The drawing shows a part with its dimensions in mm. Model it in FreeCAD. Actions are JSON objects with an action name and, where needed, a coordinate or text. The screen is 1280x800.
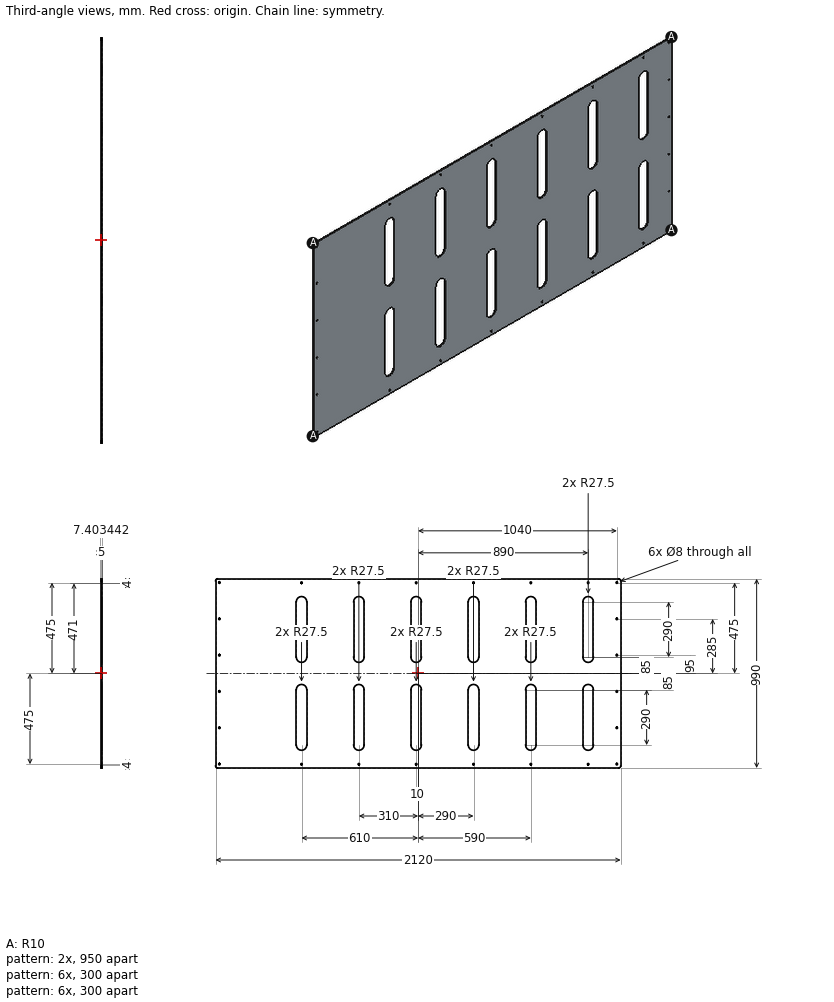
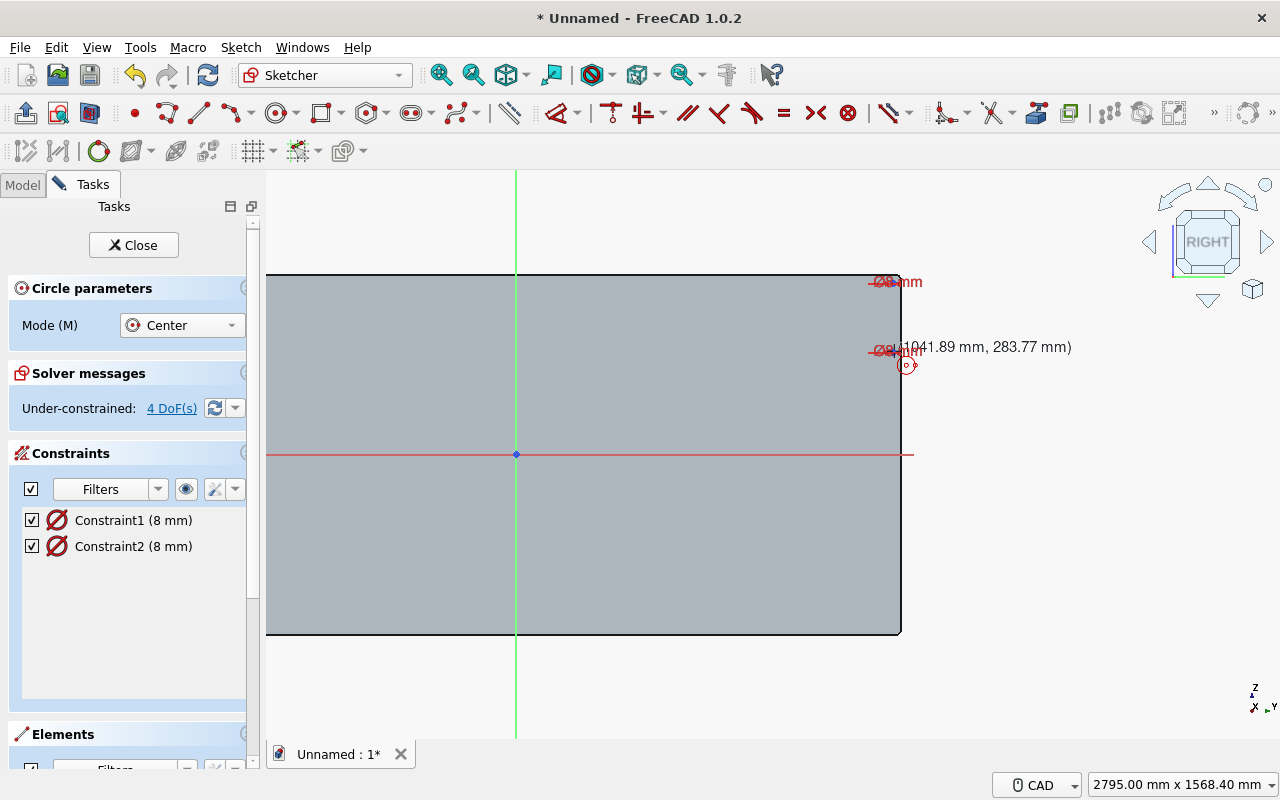
{"action": "scroll", "coordinate": [893, 420], "scroll_direction": "up", "scroll_amount": 14}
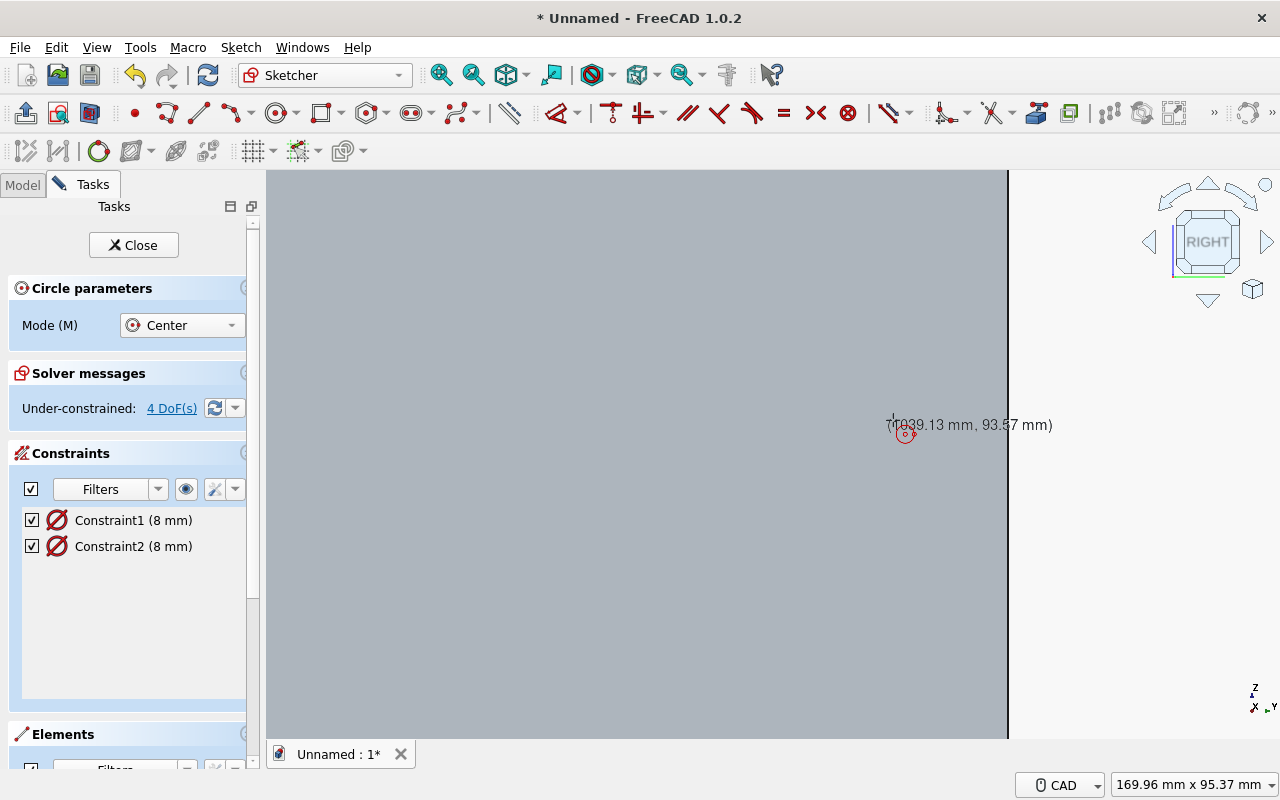
{"action": "scroll", "coordinate": [893, 420], "scroll_direction": "down", "scroll_amount": 14}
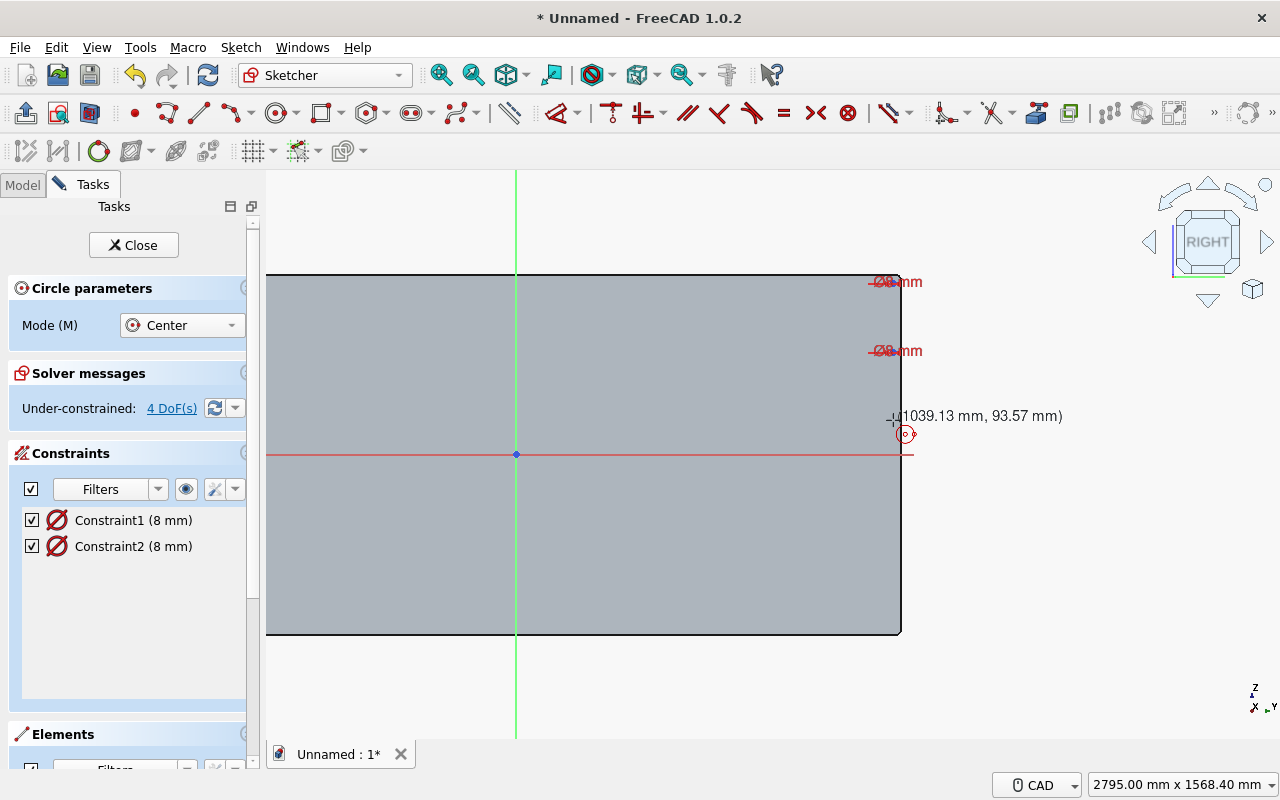
{"action": "left_click", "coordinate": [893, 420]}
{"action": "mouse_move", "coordinate": [894, 419]}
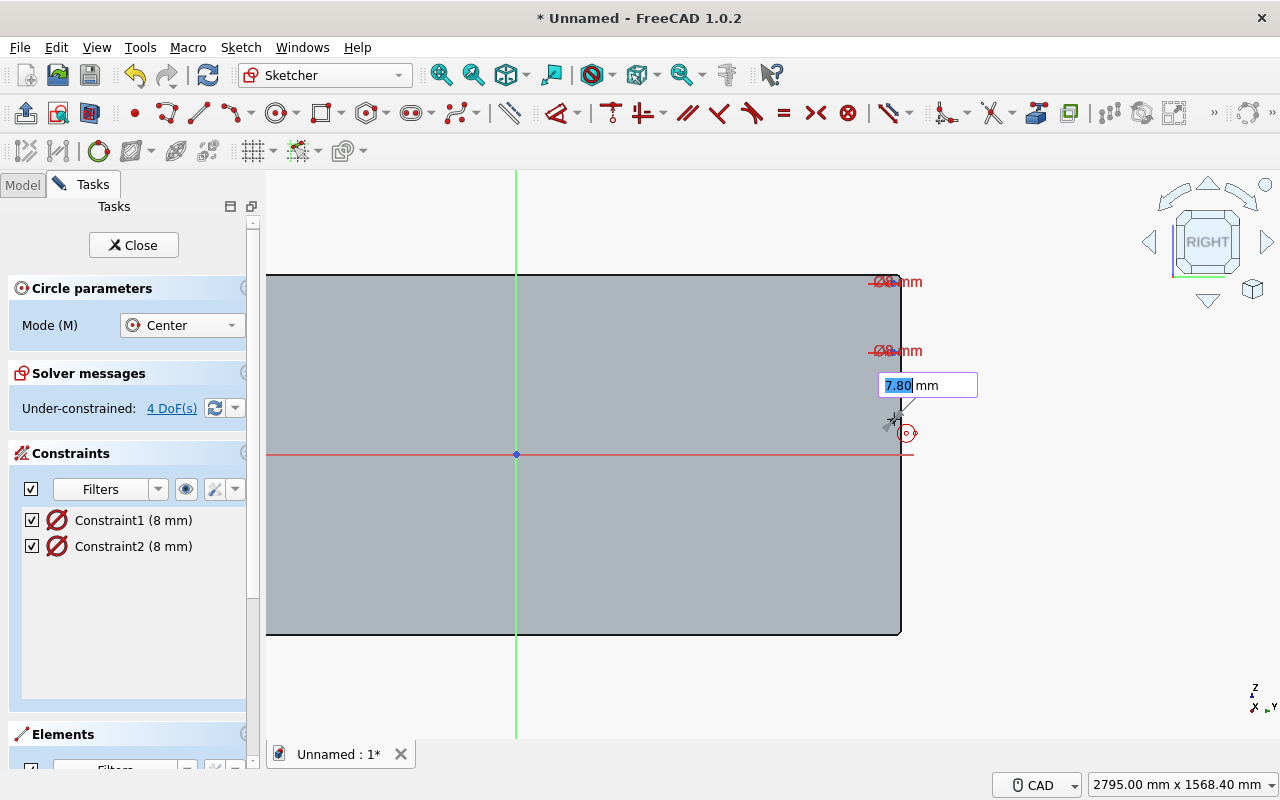
{"action": "type", "text": "8"}
{"action": "key", "text": "Return"}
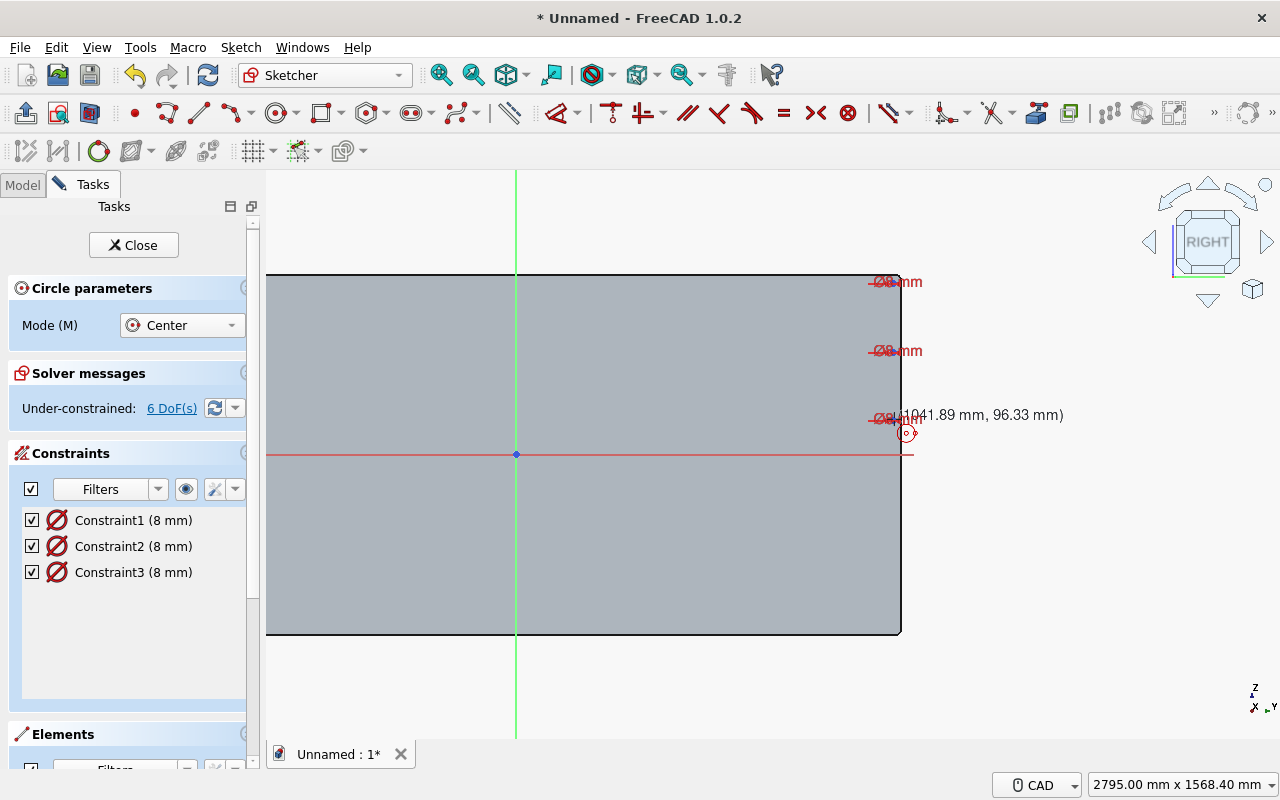
{"action": "scroll", "coordinate": [893, 489], "scroll_direction": "up", "scroll_amount": 14}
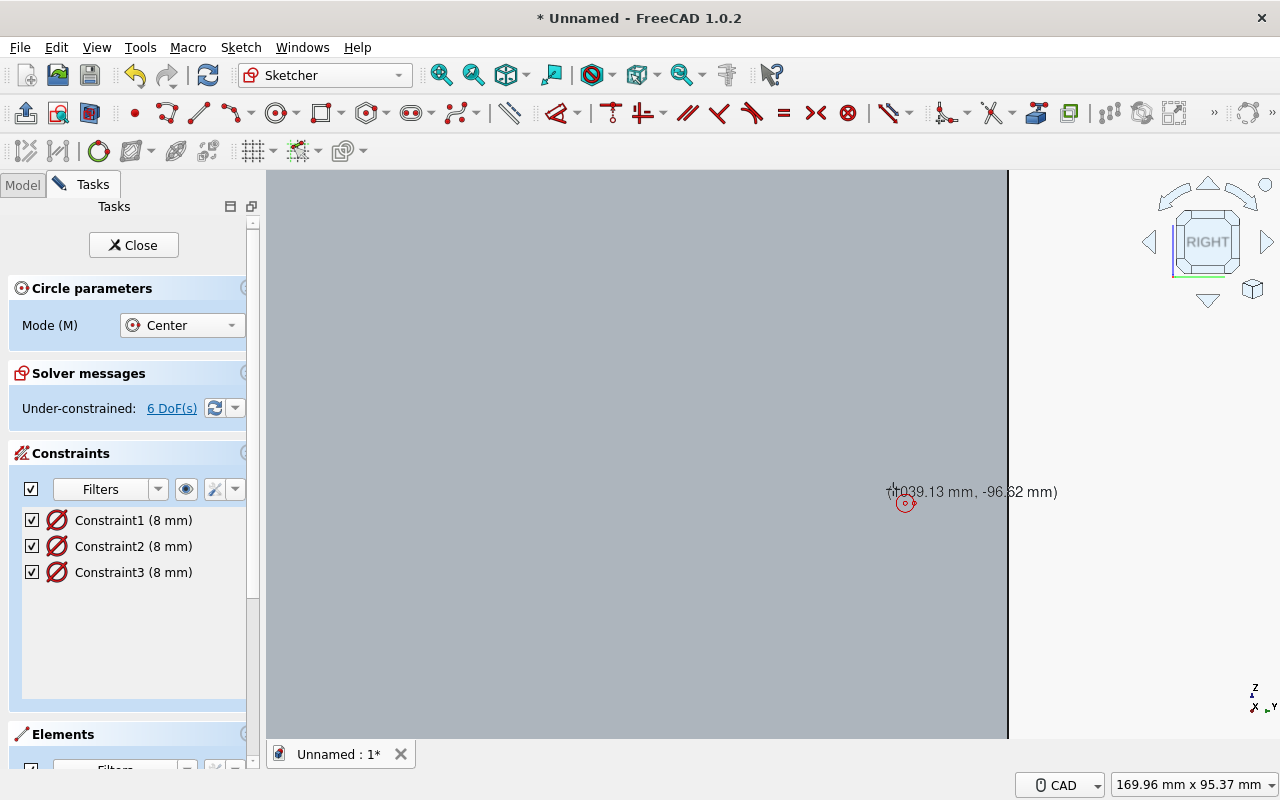
{"action": "scroll", "coordinate": [893, 489], "scroll_direction": "down", "scroll_amount": 14}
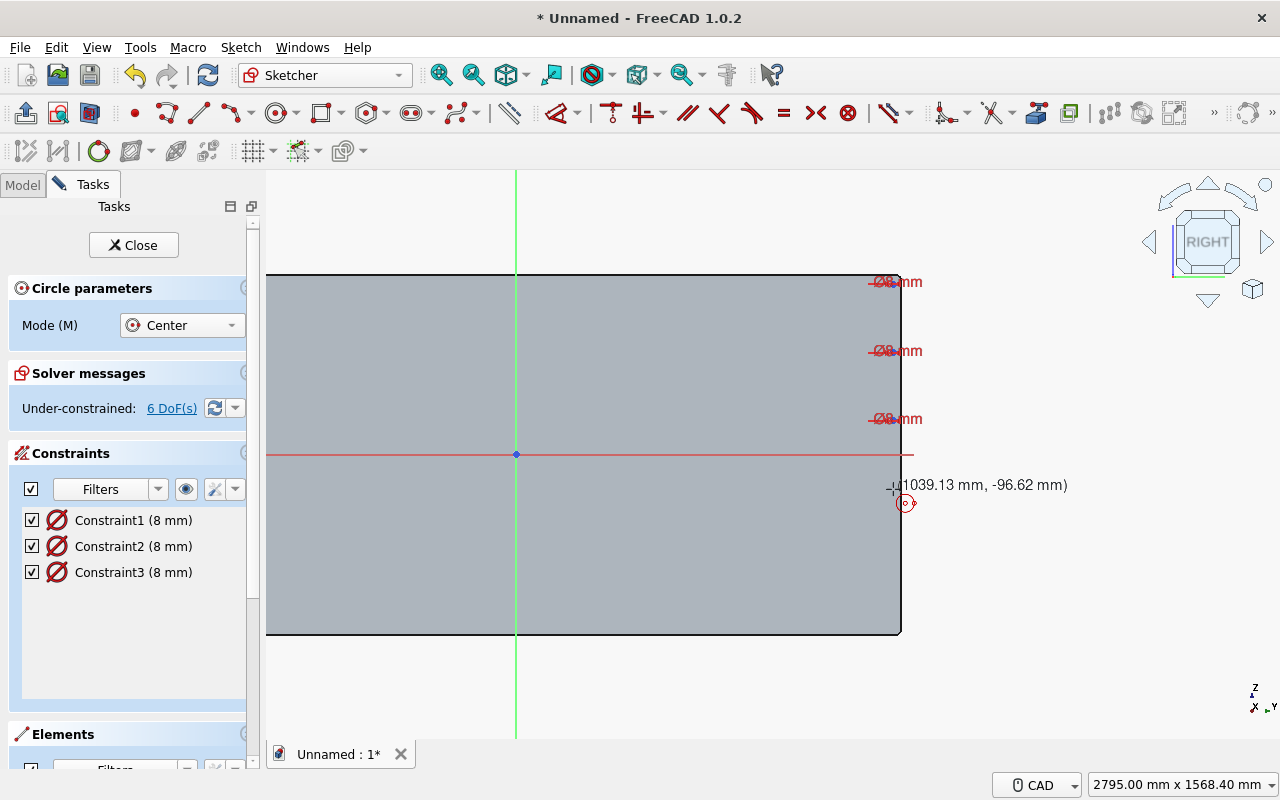
{"action": "left_click", "coordinate": [893, 489]}
{"action": "mouse_move", "coordinate": [894, 488]}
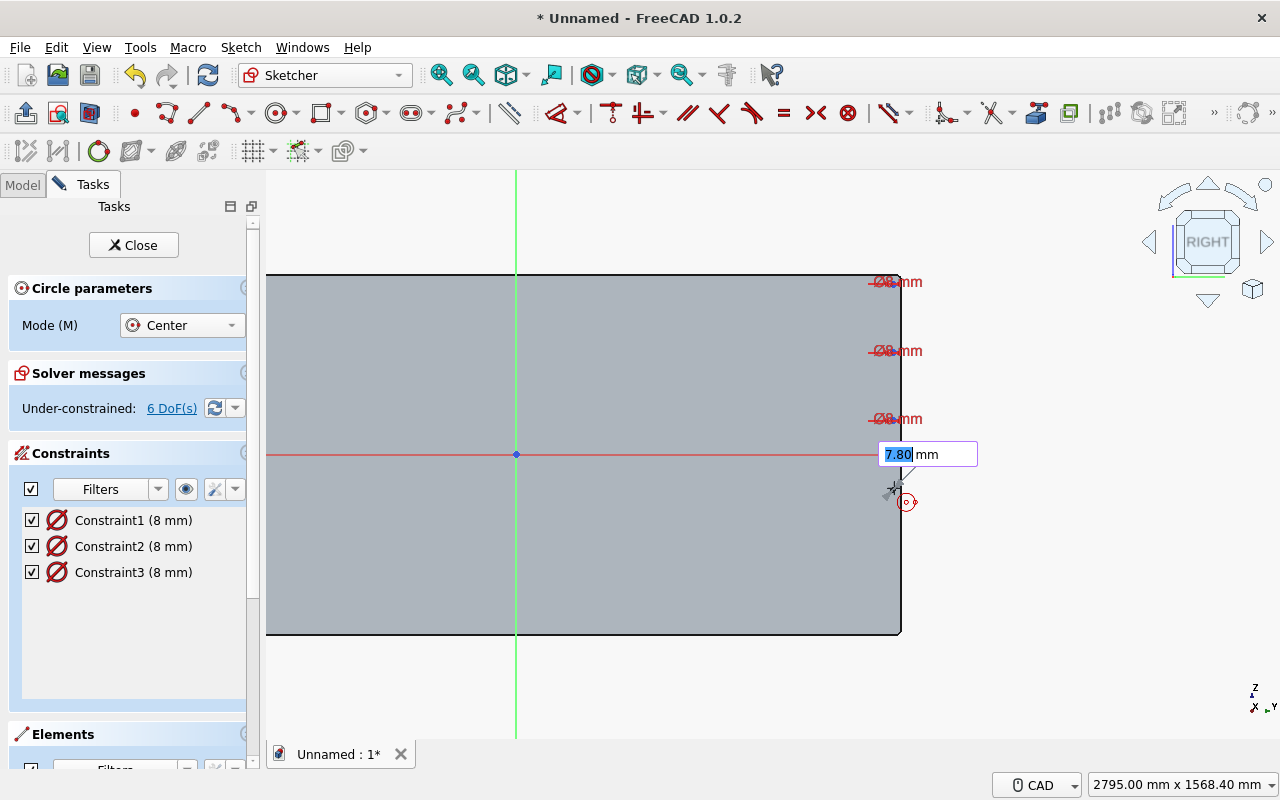
{"action": "type", "text": "8"}
{"action": "key", "text": "Return"}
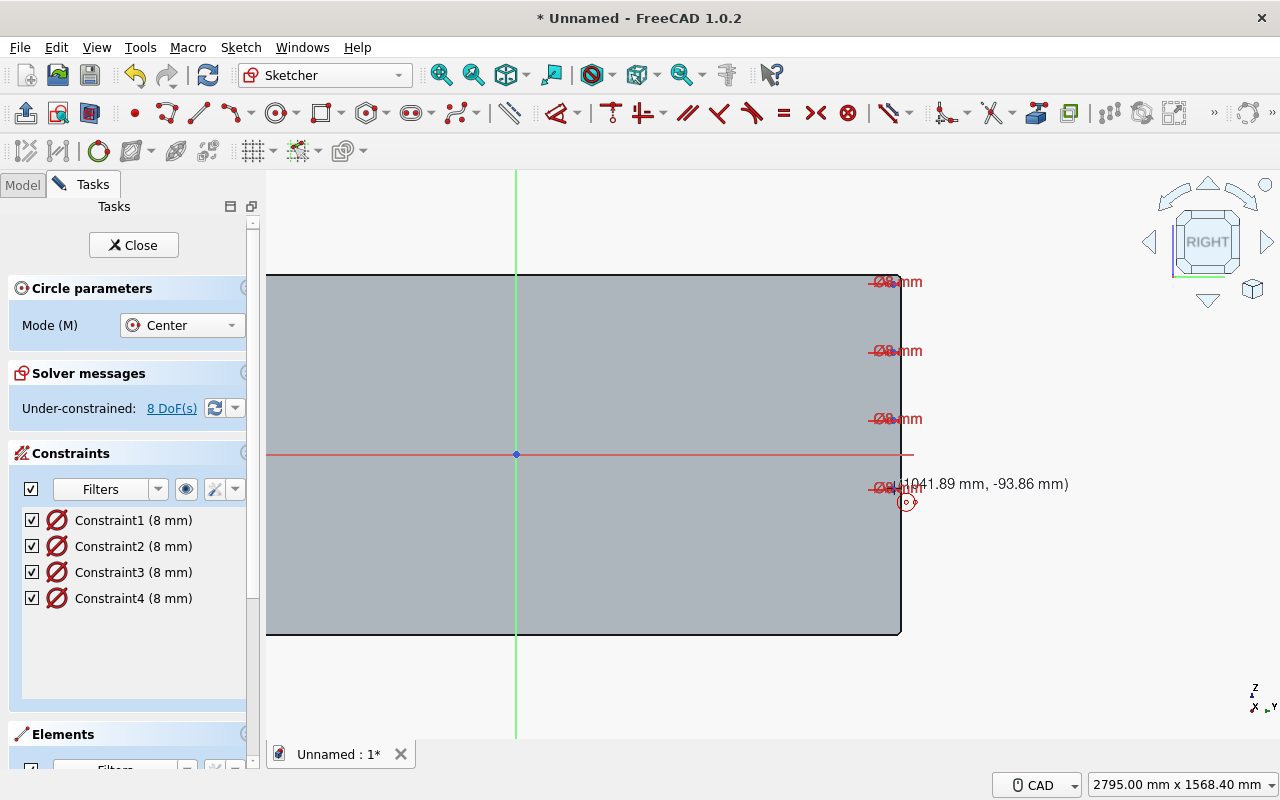
{"action": "scroll", "coordinate": [893, 558], "scroll_direction": "up", "scroll_amount": 14}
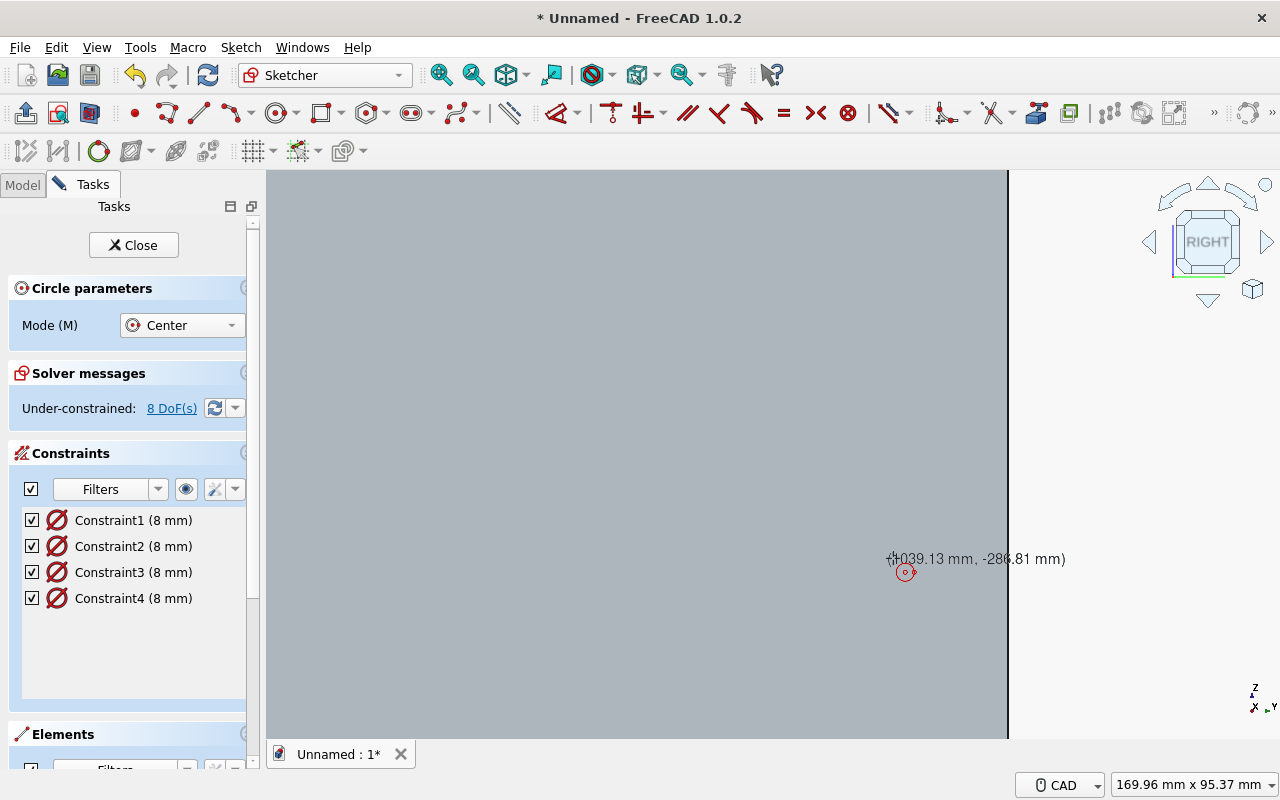
{"action": "scroll", "coordinate": [893, 558], "scroll_direction": "down", "scroll_amount": 14}